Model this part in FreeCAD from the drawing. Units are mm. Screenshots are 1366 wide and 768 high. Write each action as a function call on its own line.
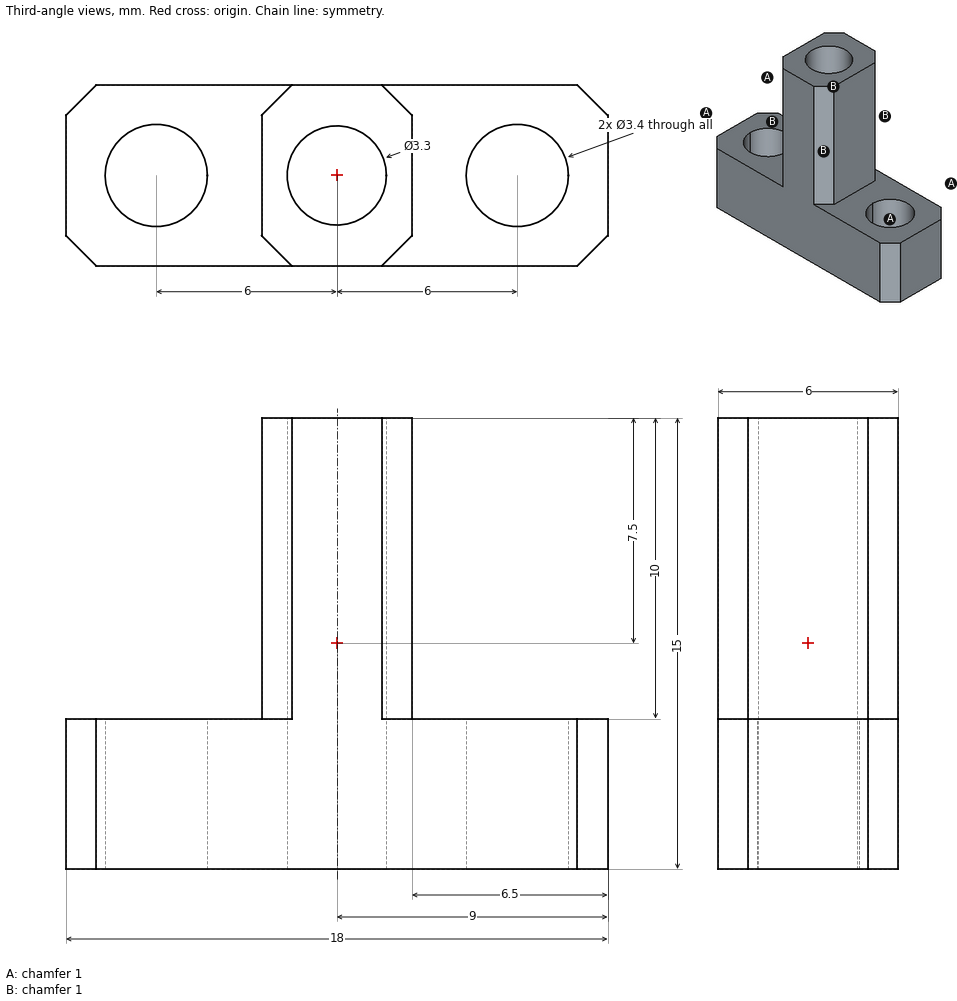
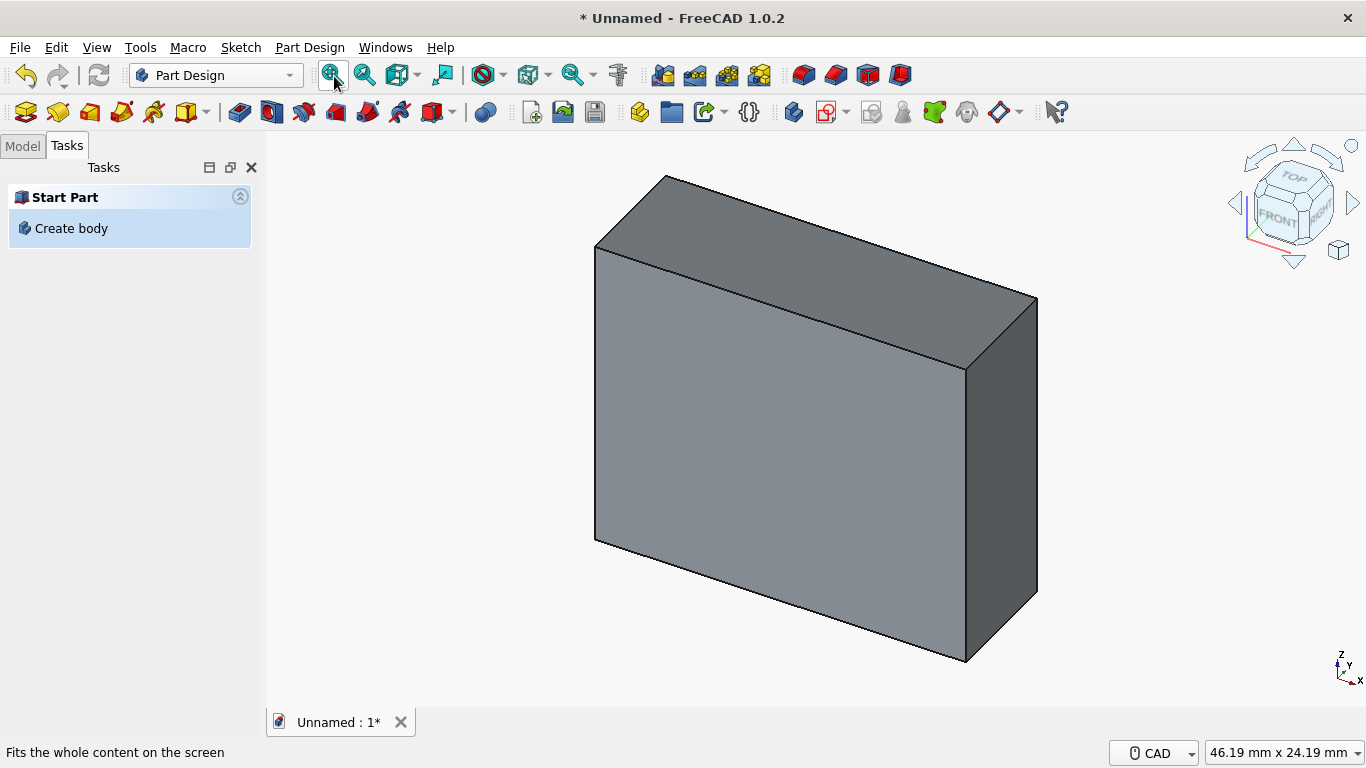
key(5)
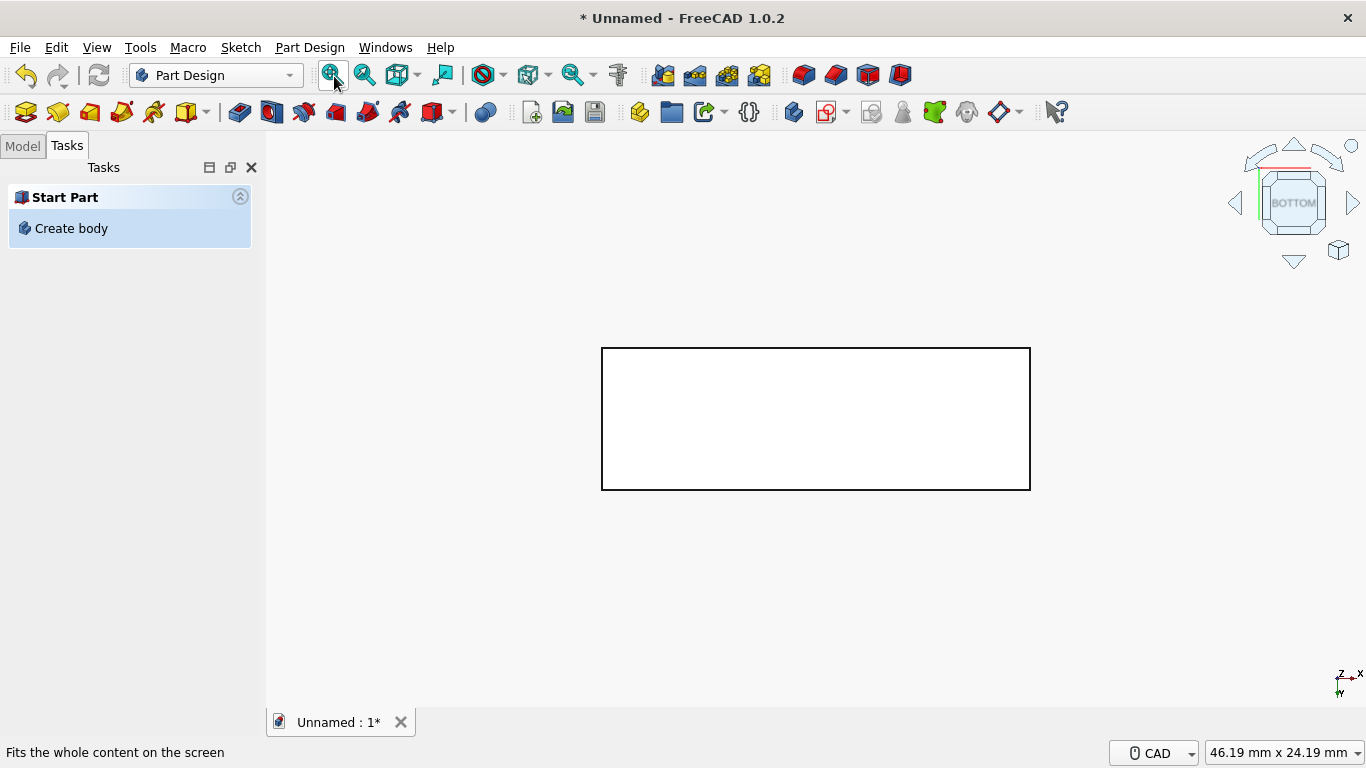
click(334, 76)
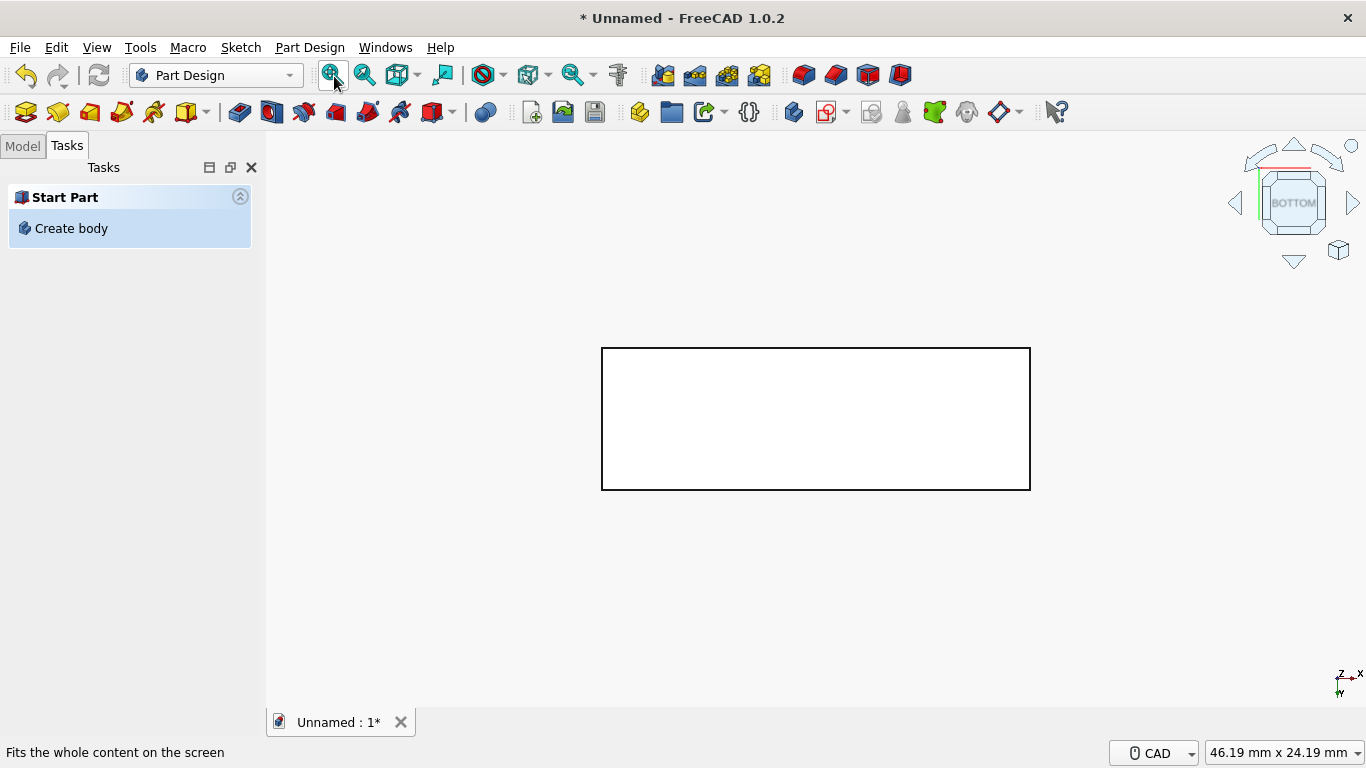
click(938, 418)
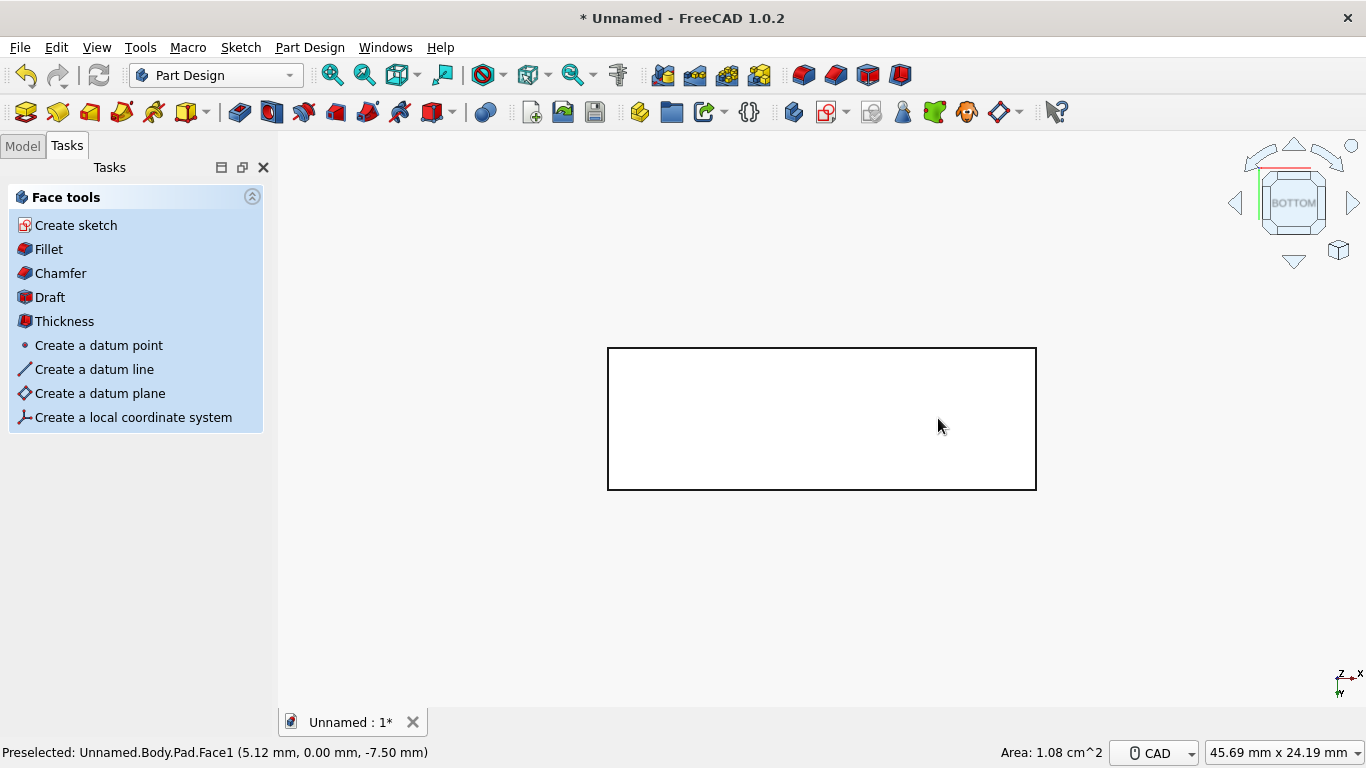
click(826, 112)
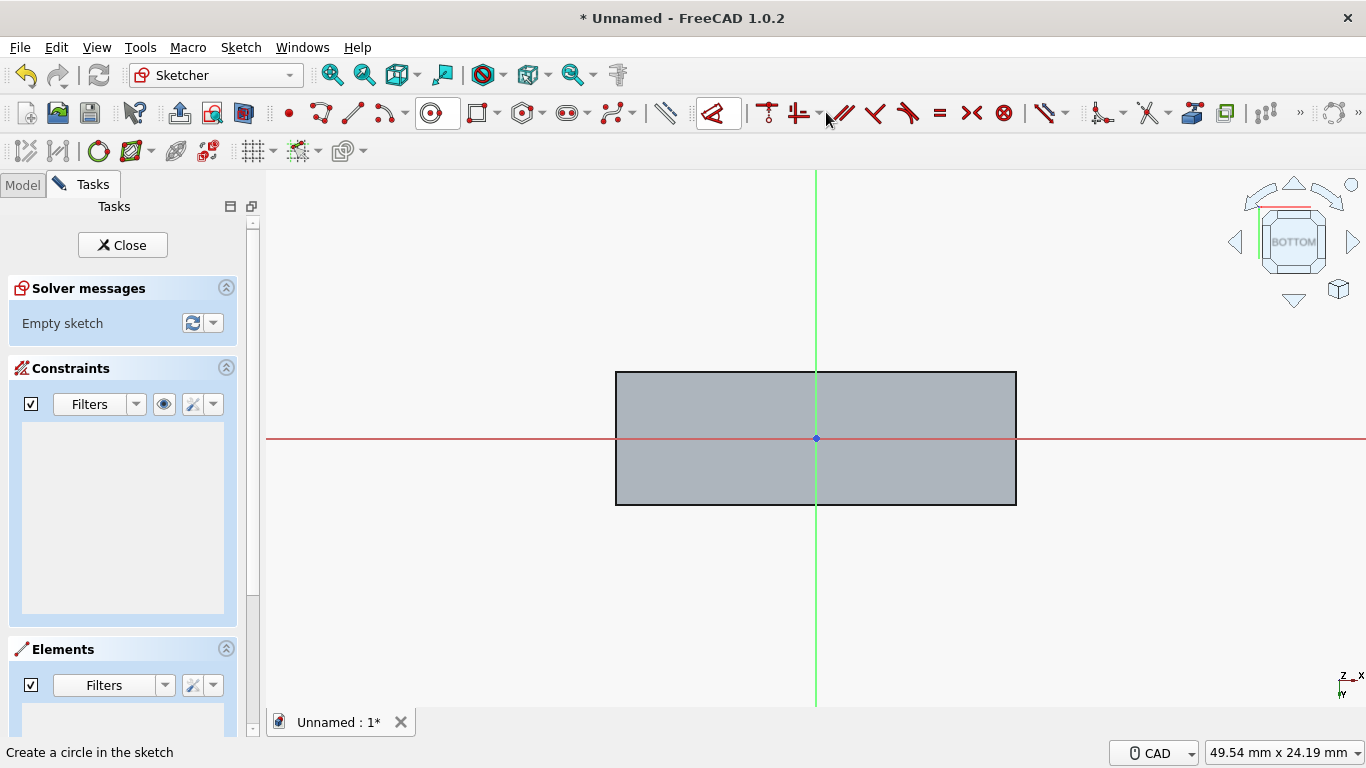
scroll(899, 438, up, 3)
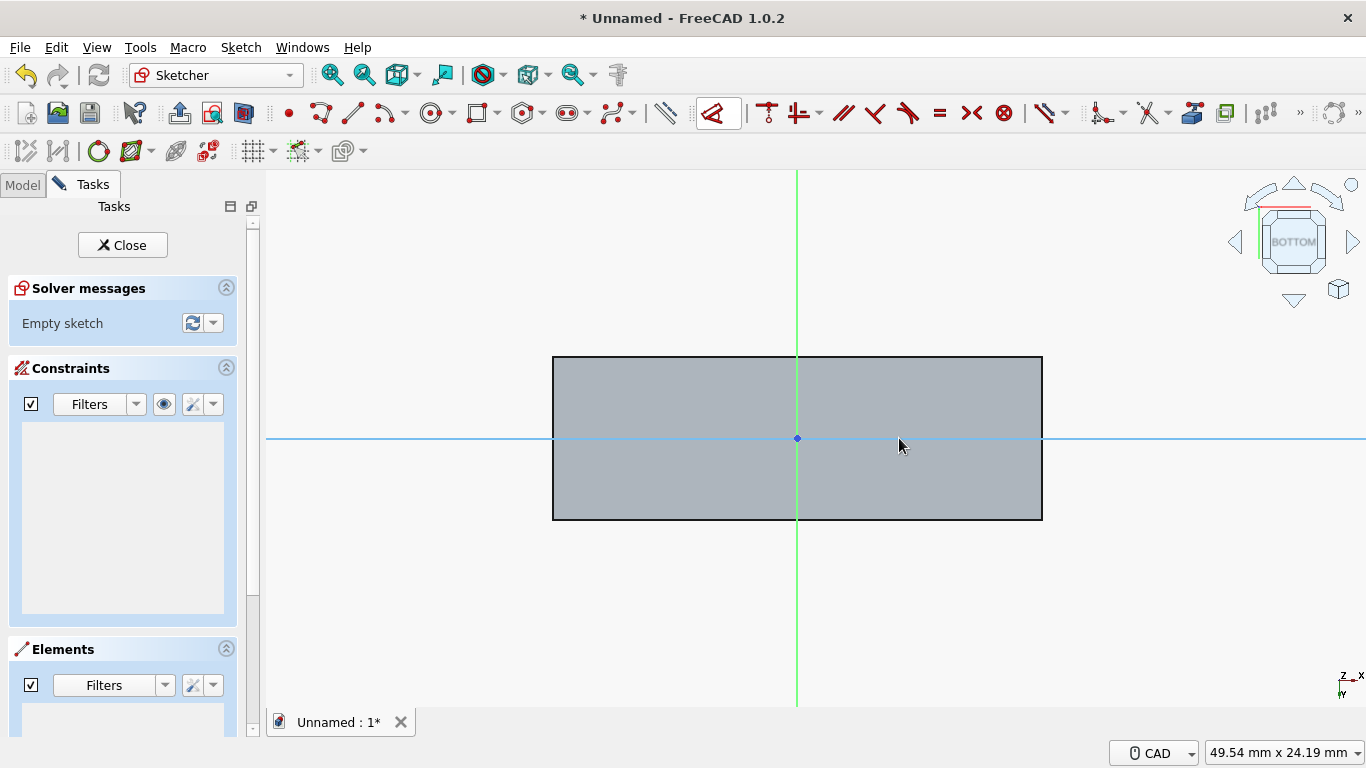
click(432, 114)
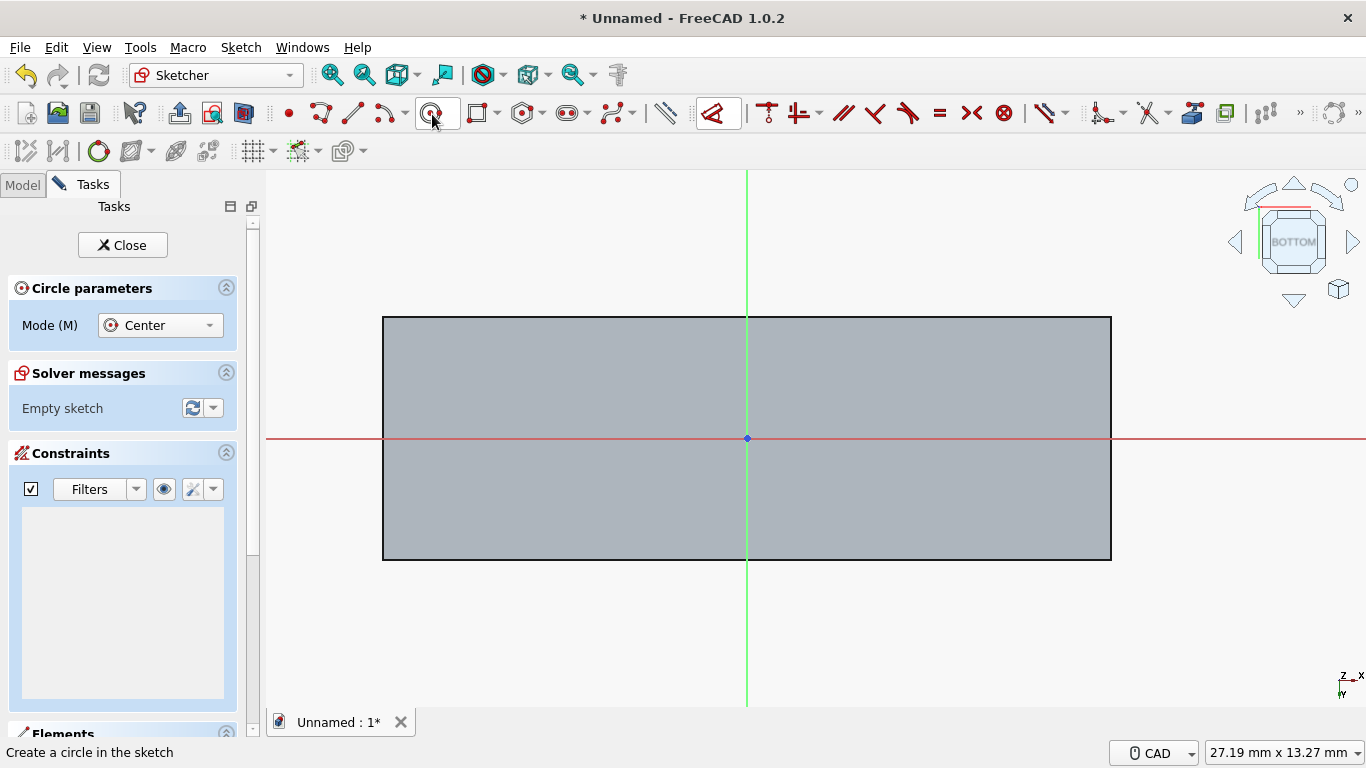
click(990, 438)
click(1039, 390)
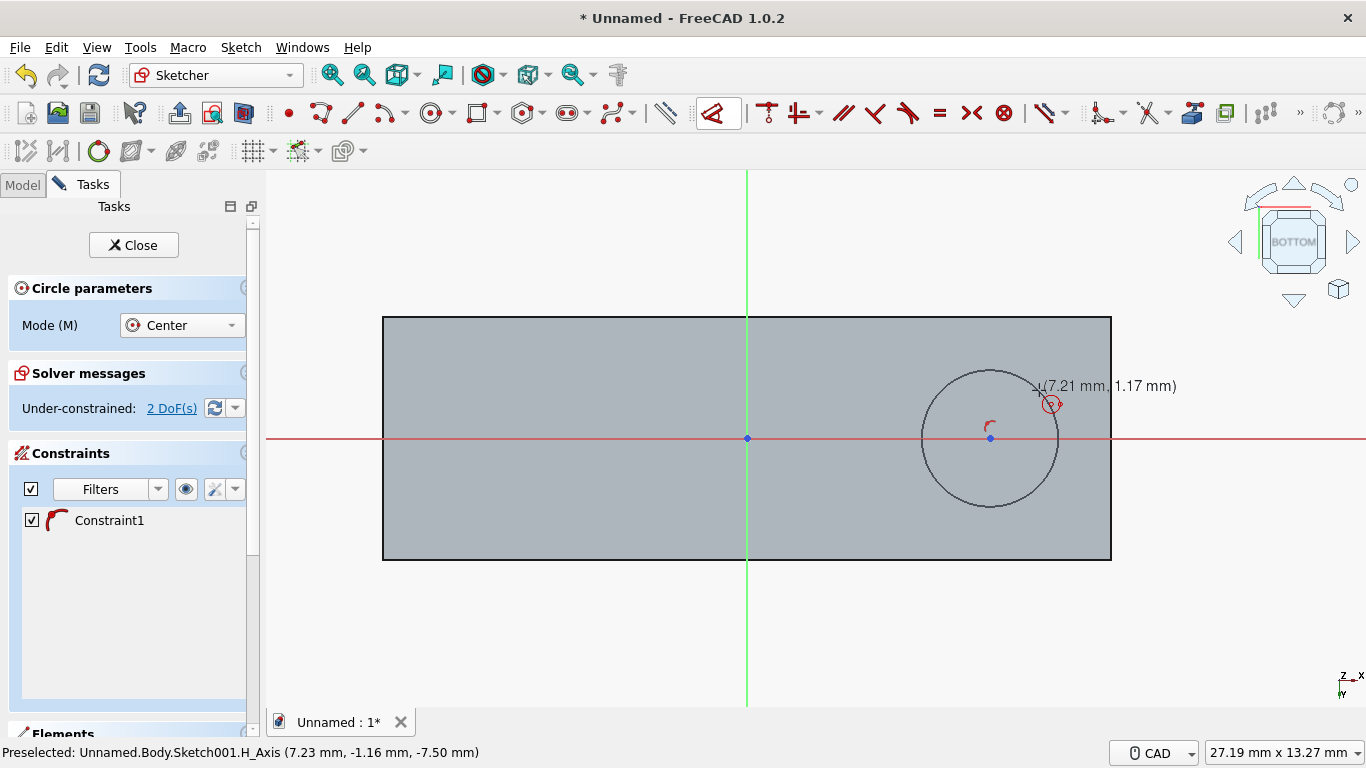
click(505, 438)
click(553, 390)
key(Escape)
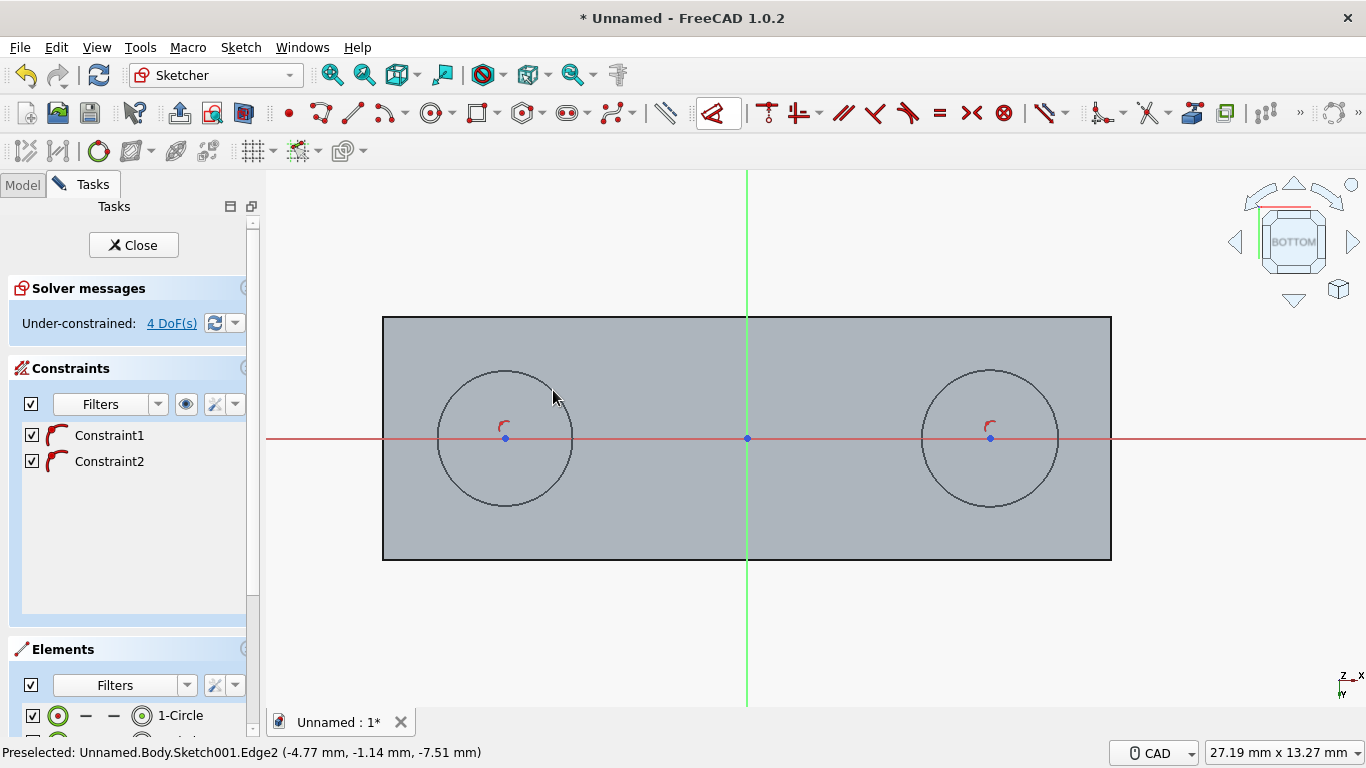
click(1038, 390)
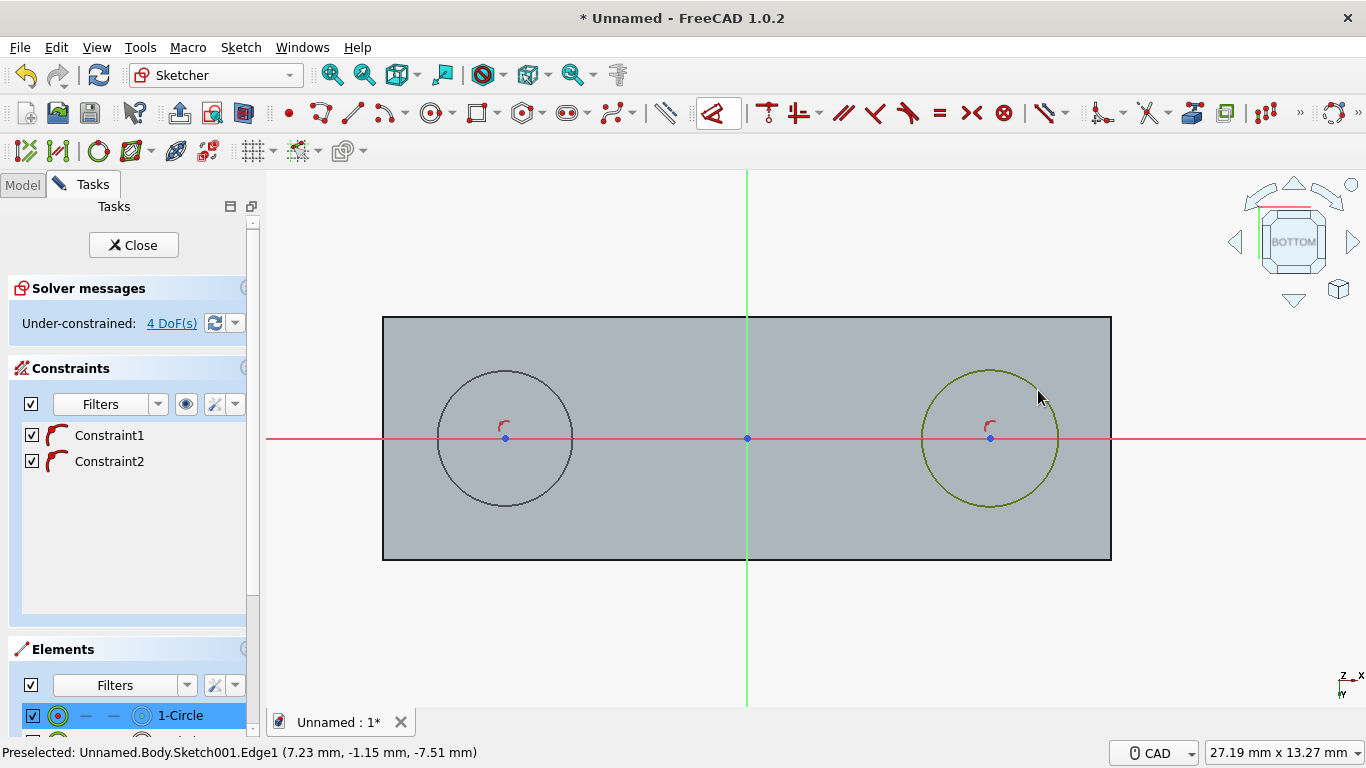
click(553, 391)